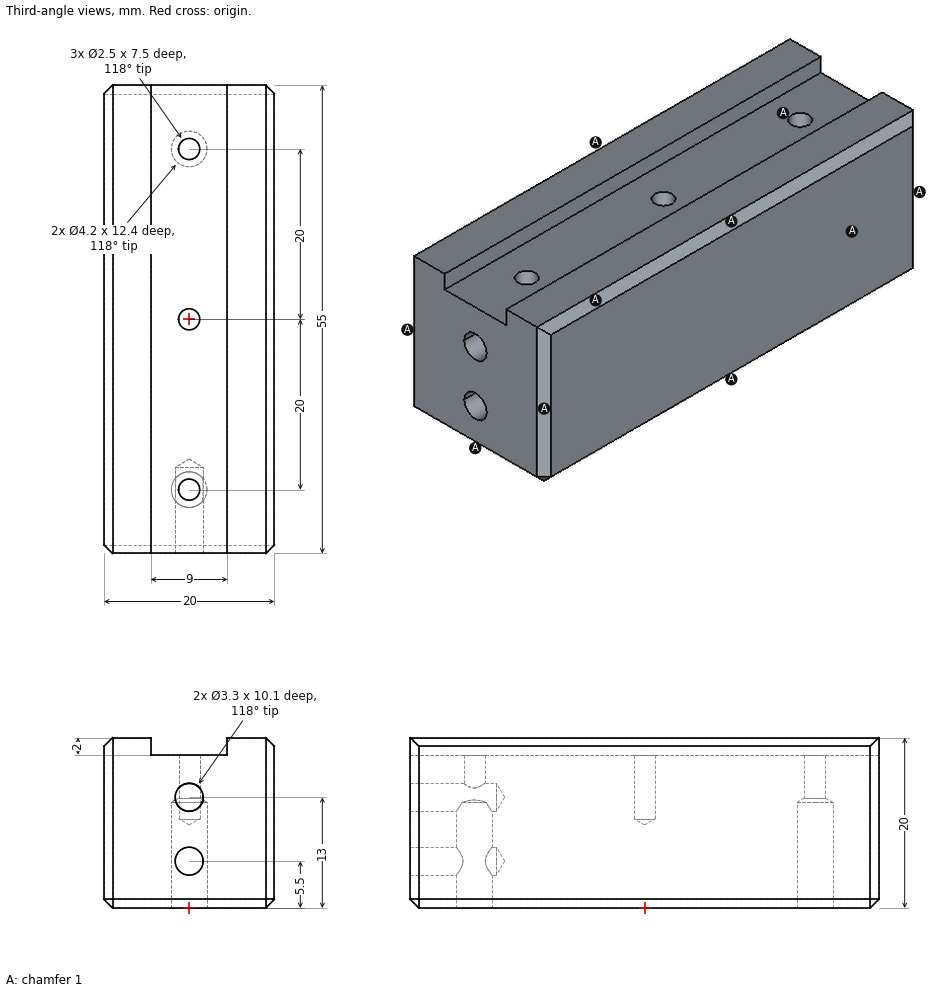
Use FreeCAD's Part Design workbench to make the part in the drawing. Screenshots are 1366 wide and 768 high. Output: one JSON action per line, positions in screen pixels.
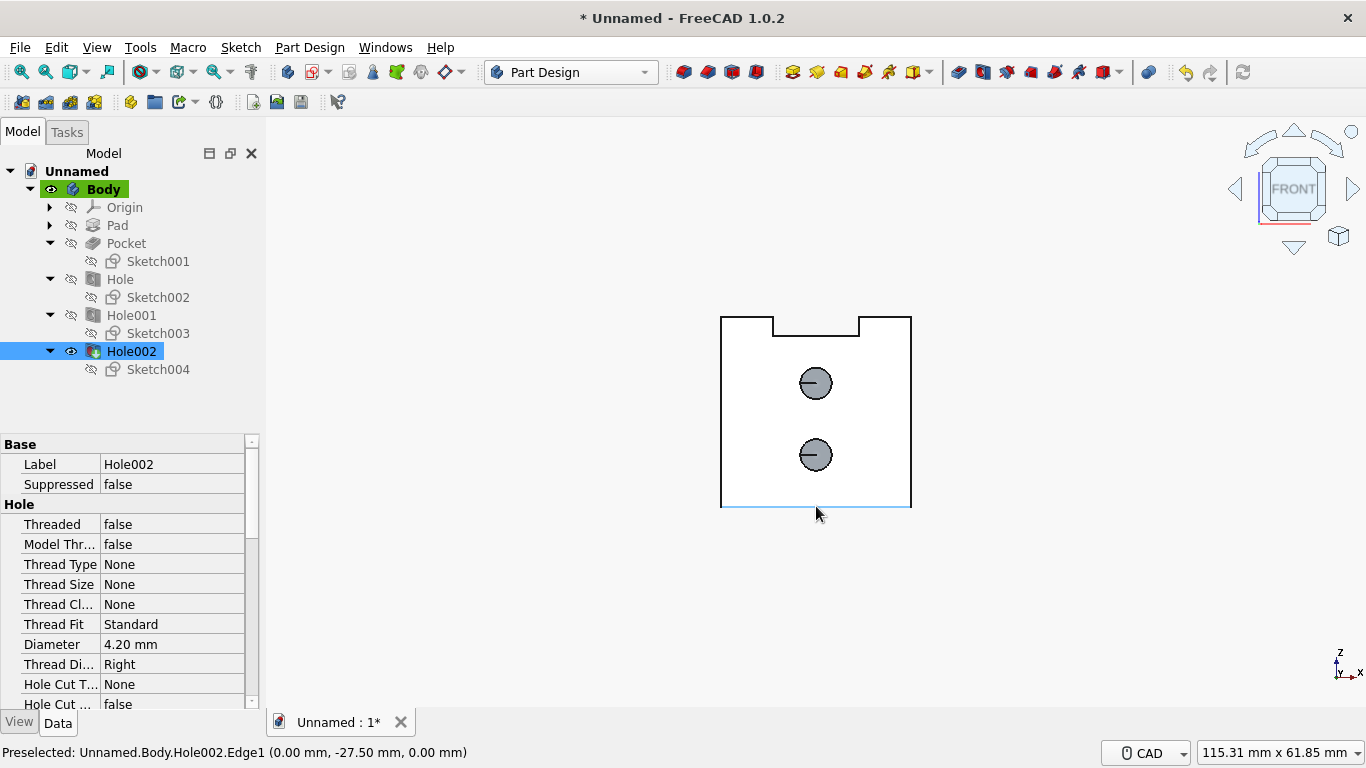
{"action": "key", "text": "3"}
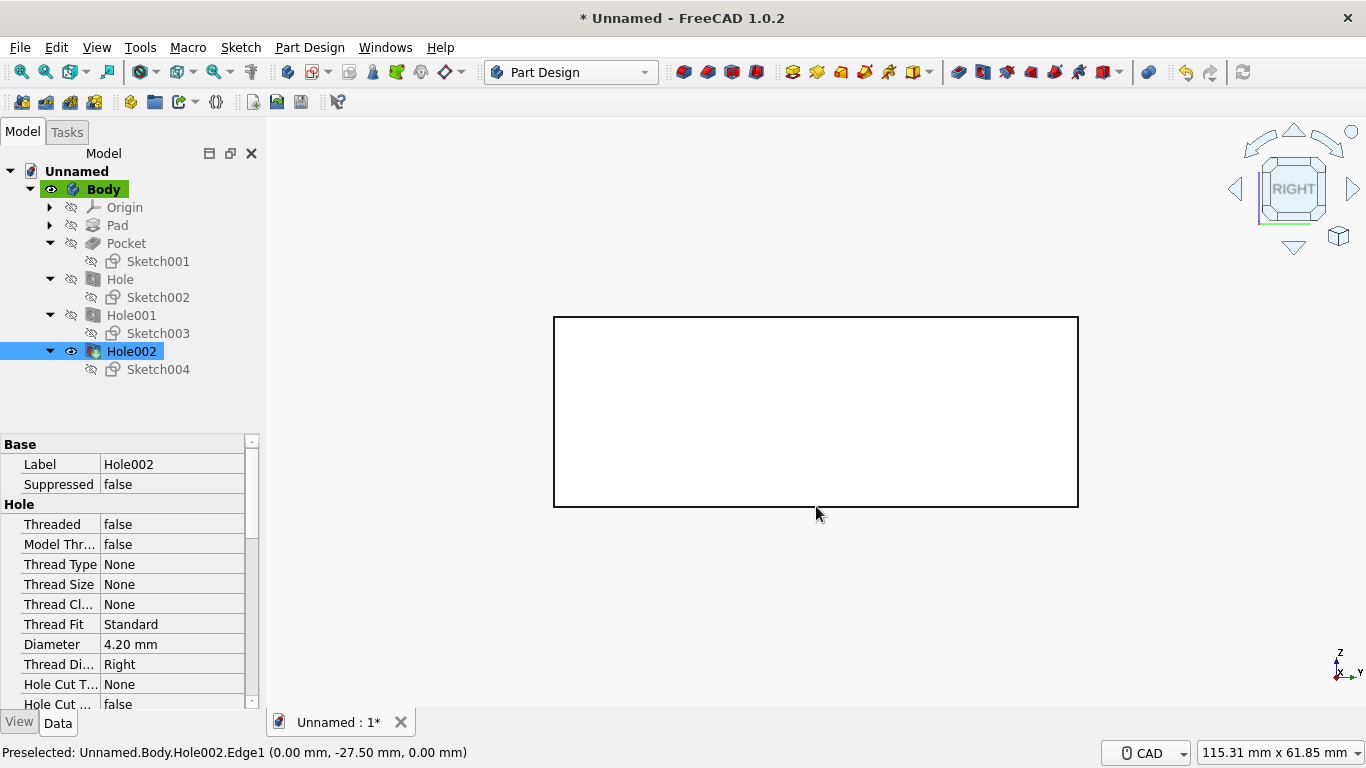
{"action": "key", "text": "5"}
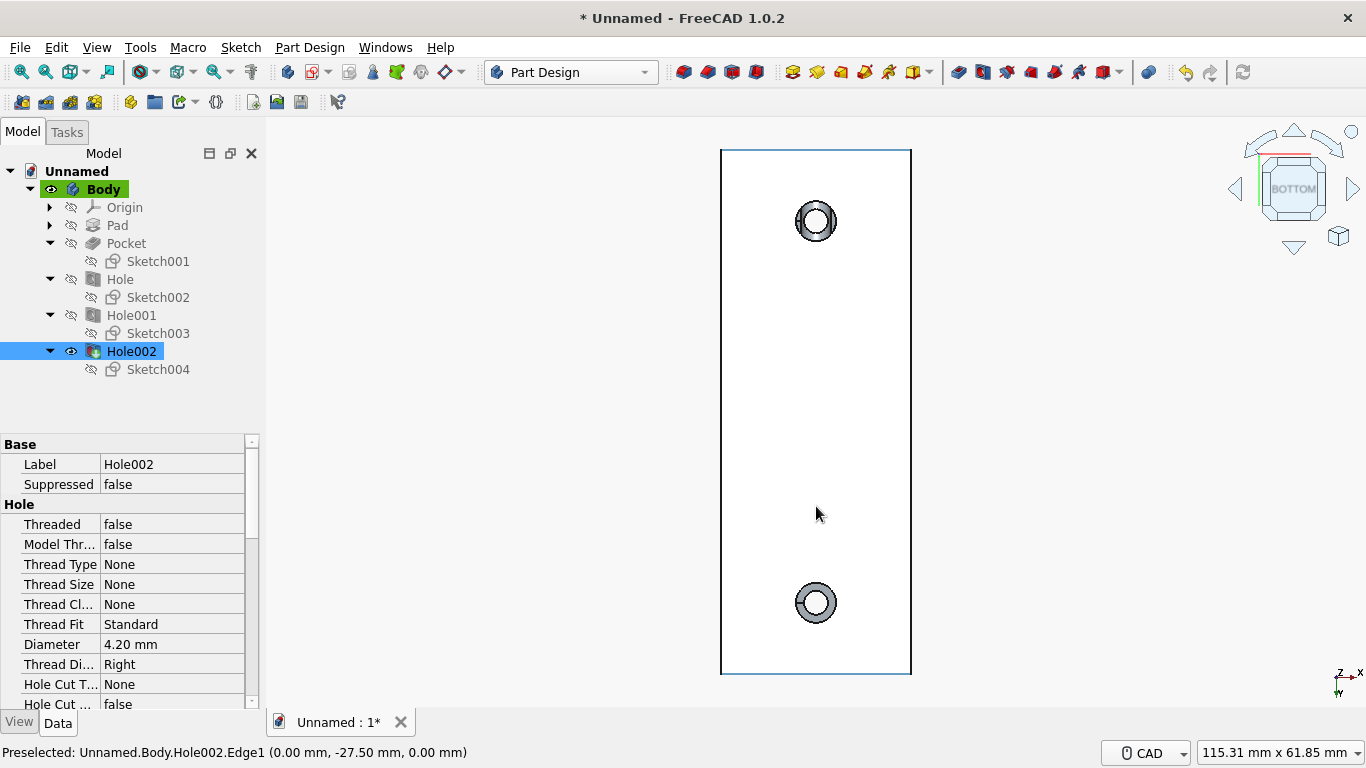
{"action": "key", "text": "4"}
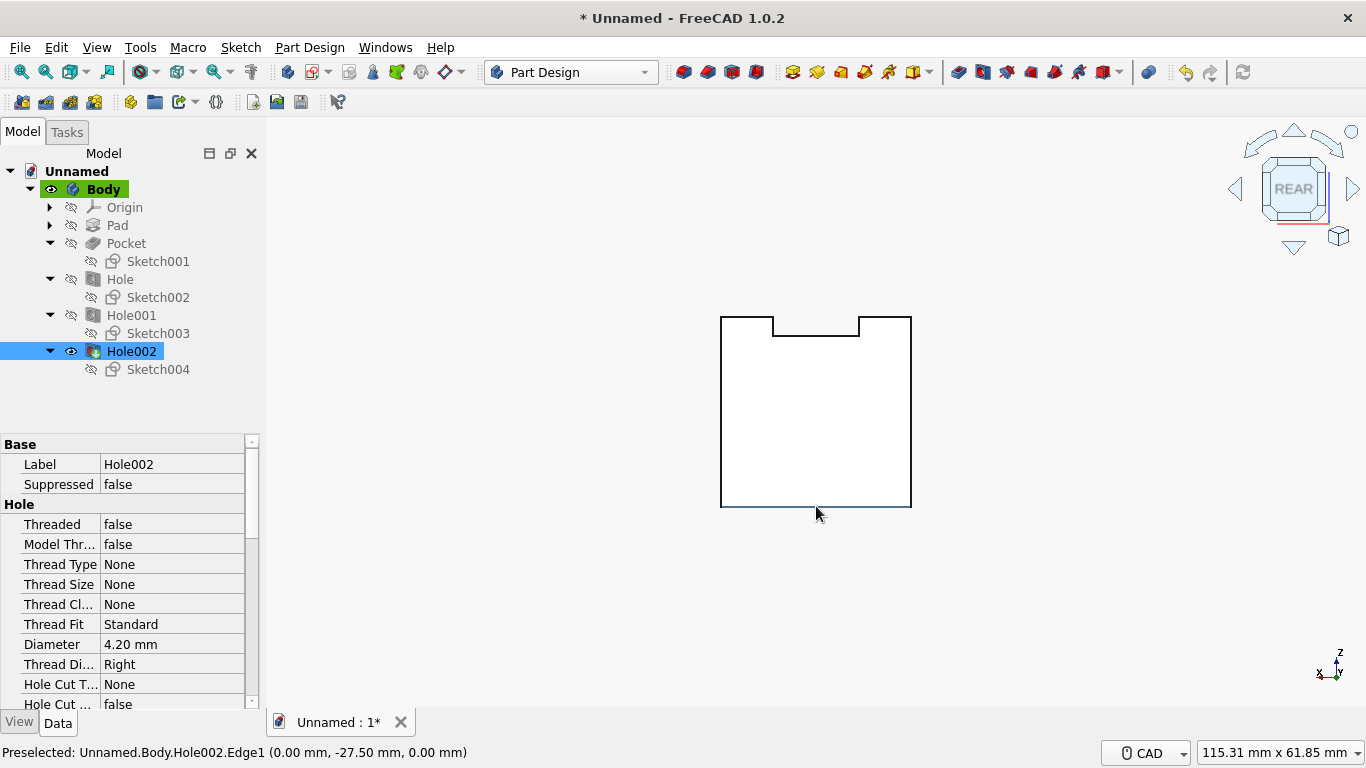
{"action": "left_click", "coordinate": [22, 72]}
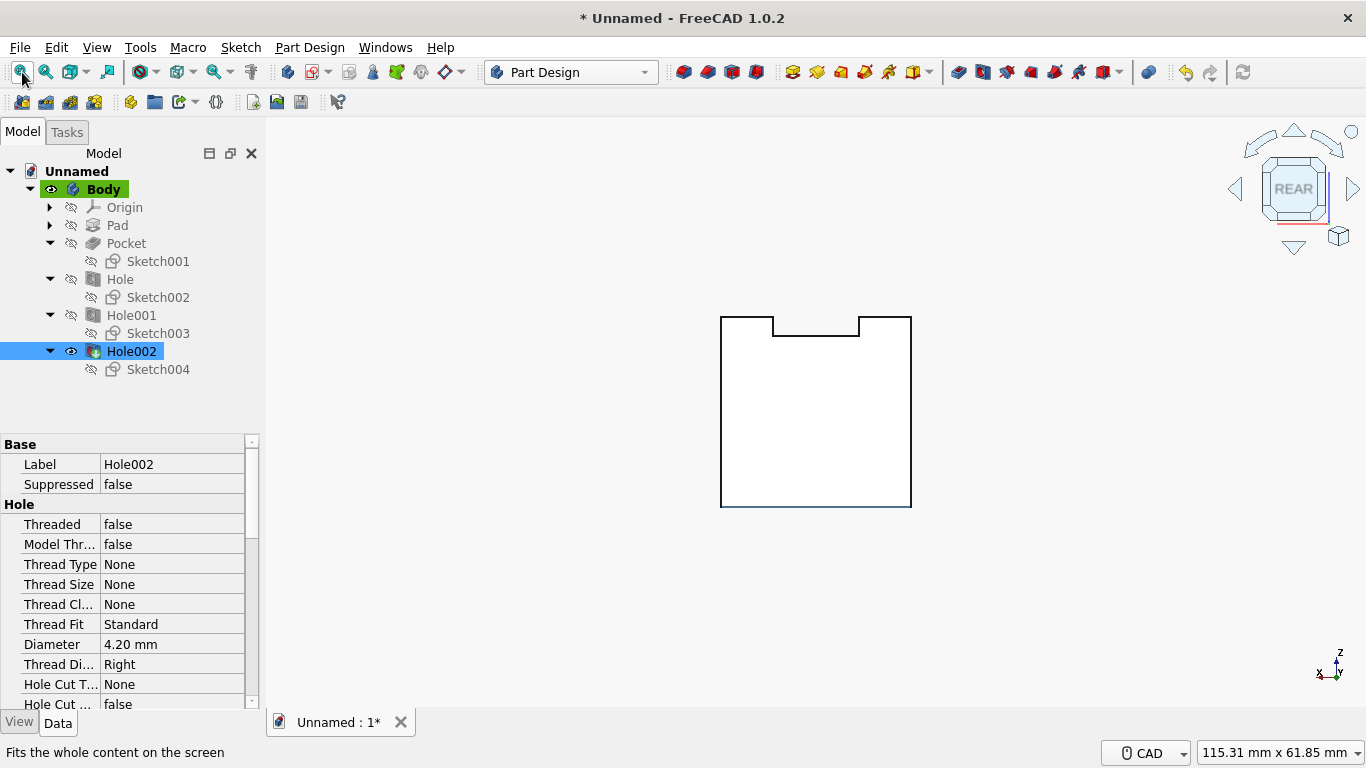
{"action": "key", "text": "6"}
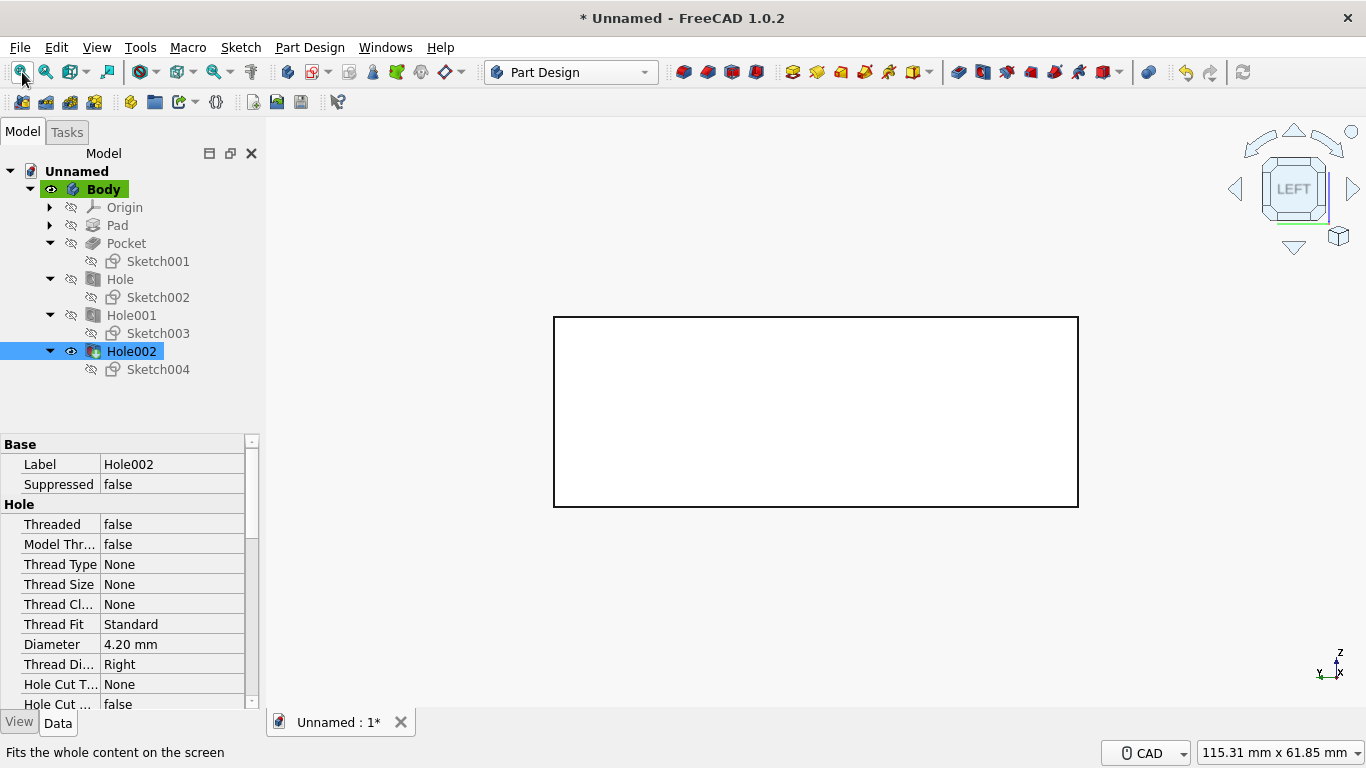
{"action": "left_click", "coordinate": [666, 411], "text": "ctrl"}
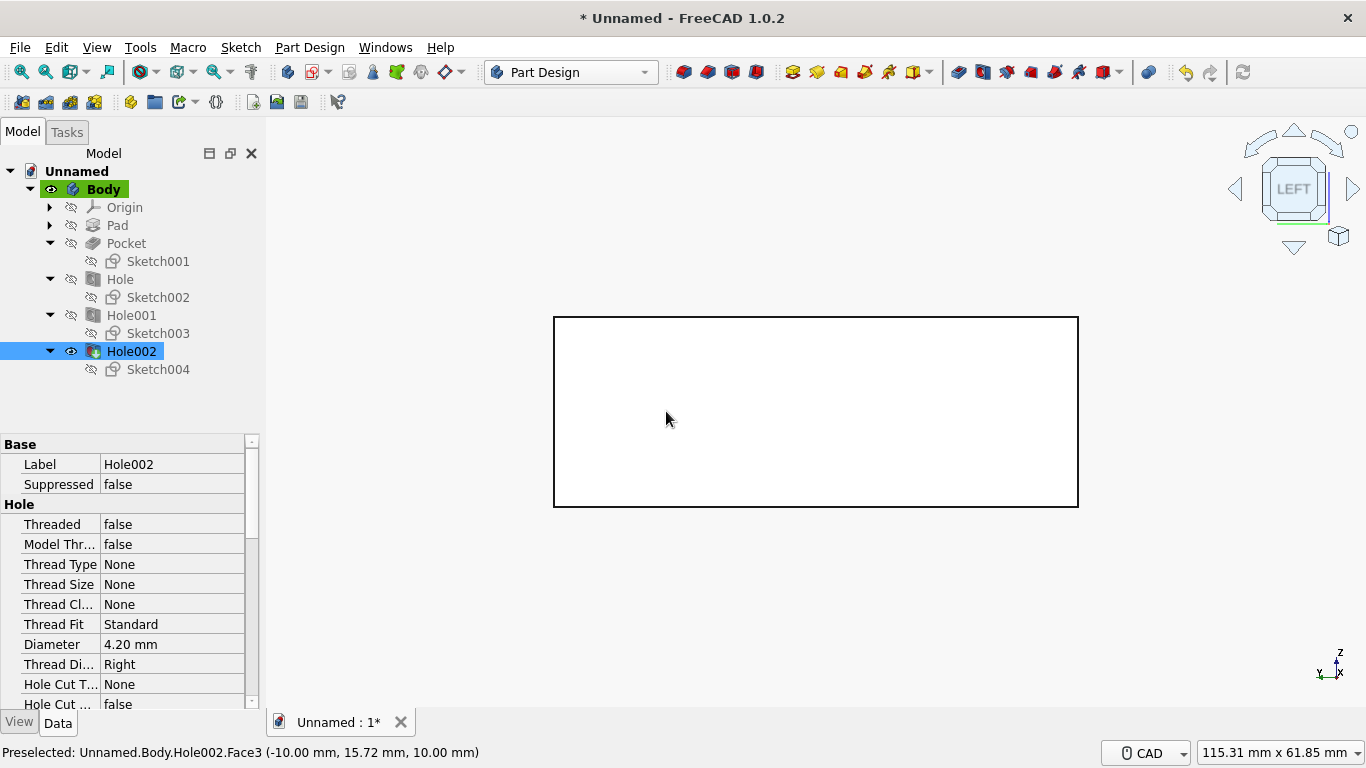
{"action": "left_click", "coordinate": [708, 72]}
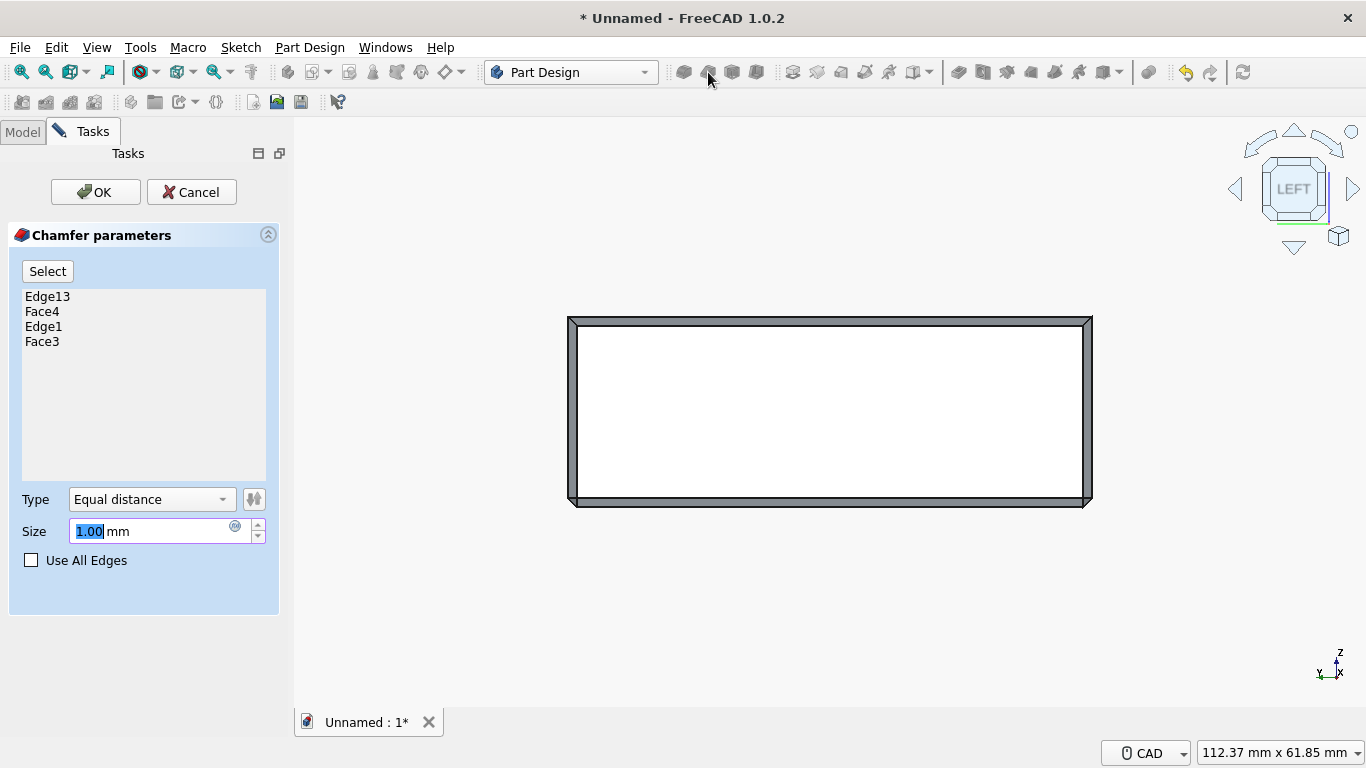
{"action": "type", "text": "1"}
{"action": "key", "text": "Tab"}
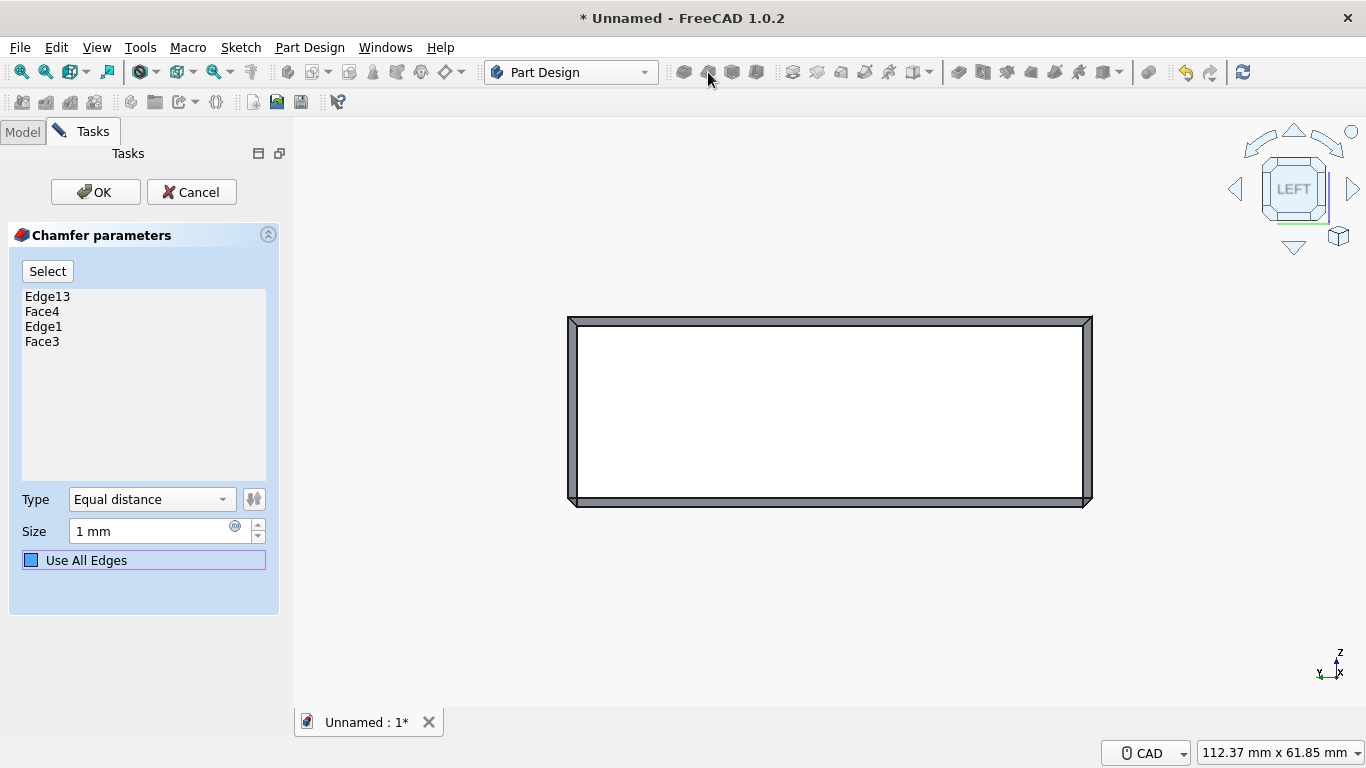
{"action": "left_click", "coordinate": [96, 192]}